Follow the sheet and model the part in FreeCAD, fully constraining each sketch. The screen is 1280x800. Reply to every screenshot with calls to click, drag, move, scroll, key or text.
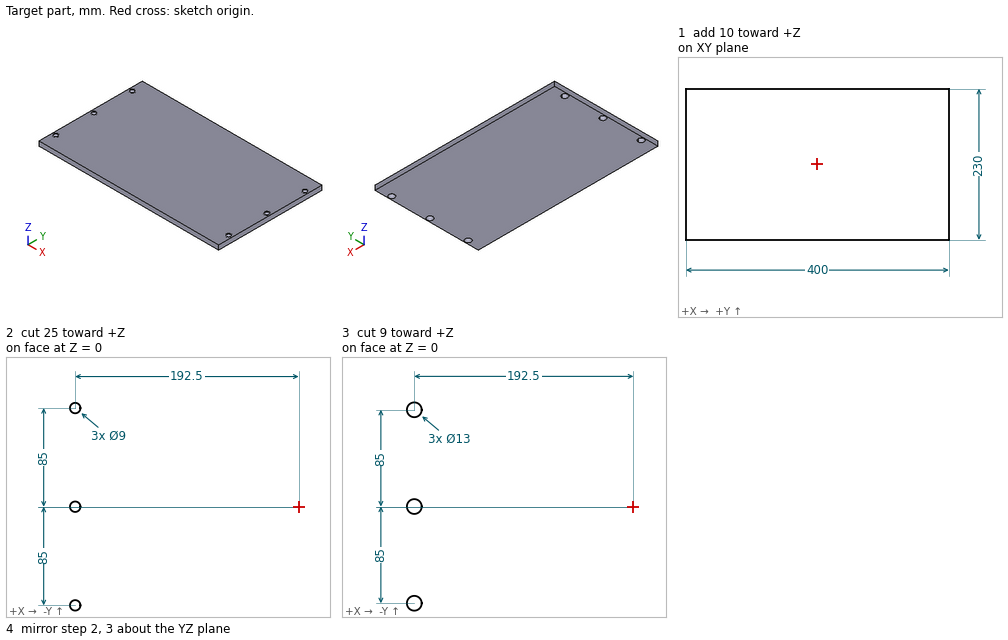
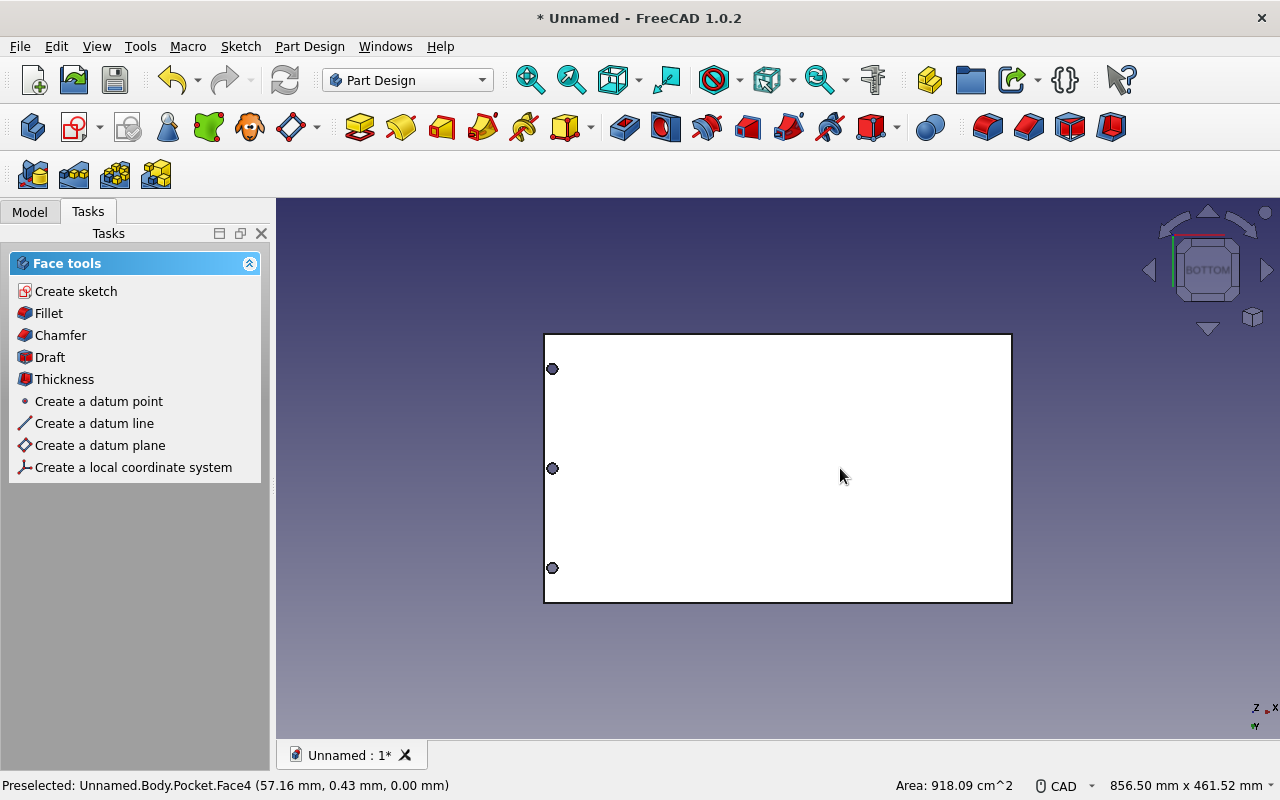
click(74, 128)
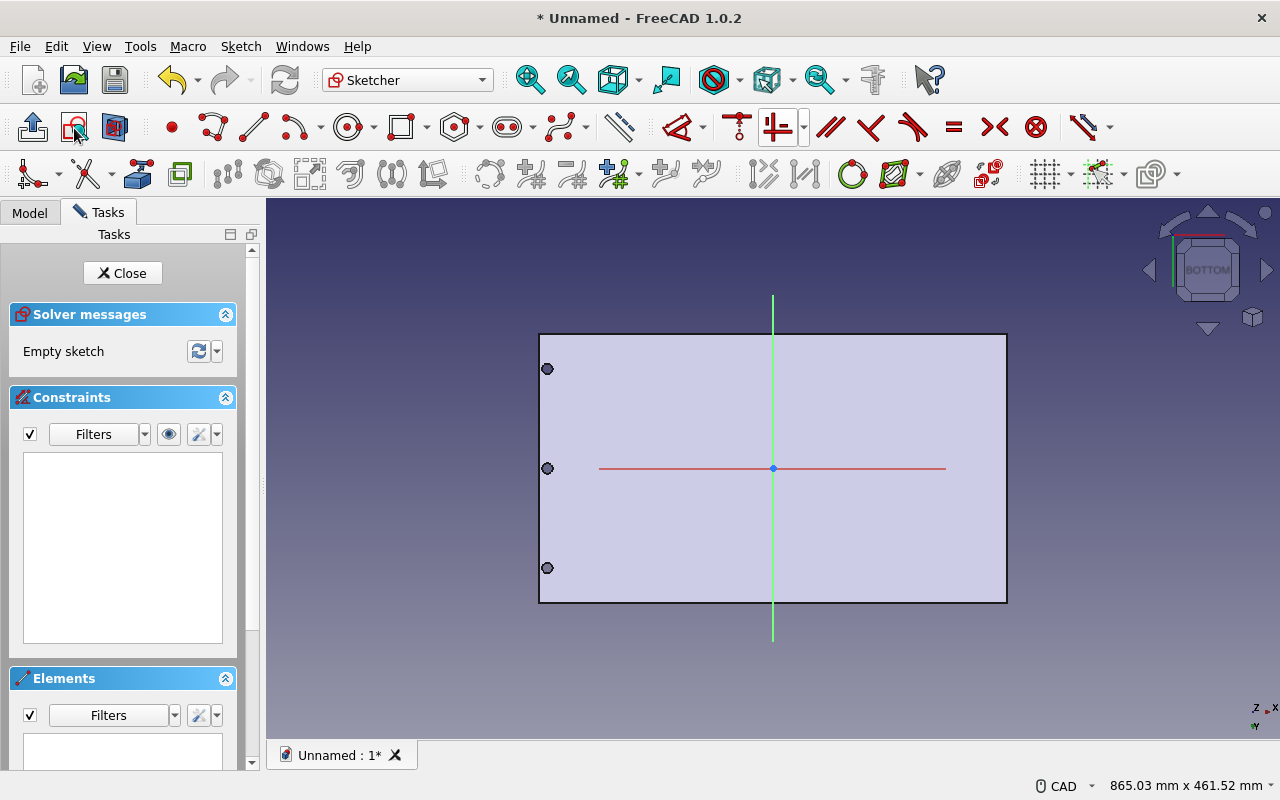
scroll(558, 469, up, 2)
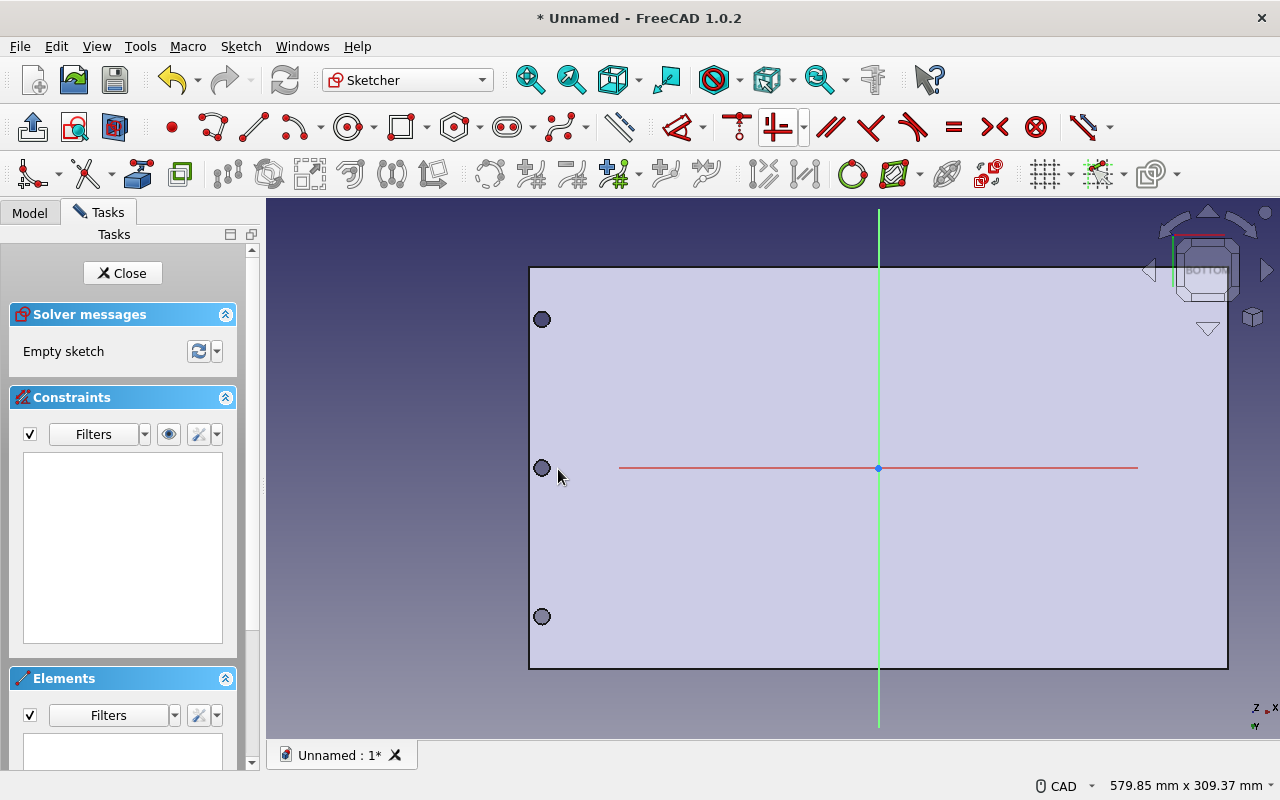
key(g)
key(c)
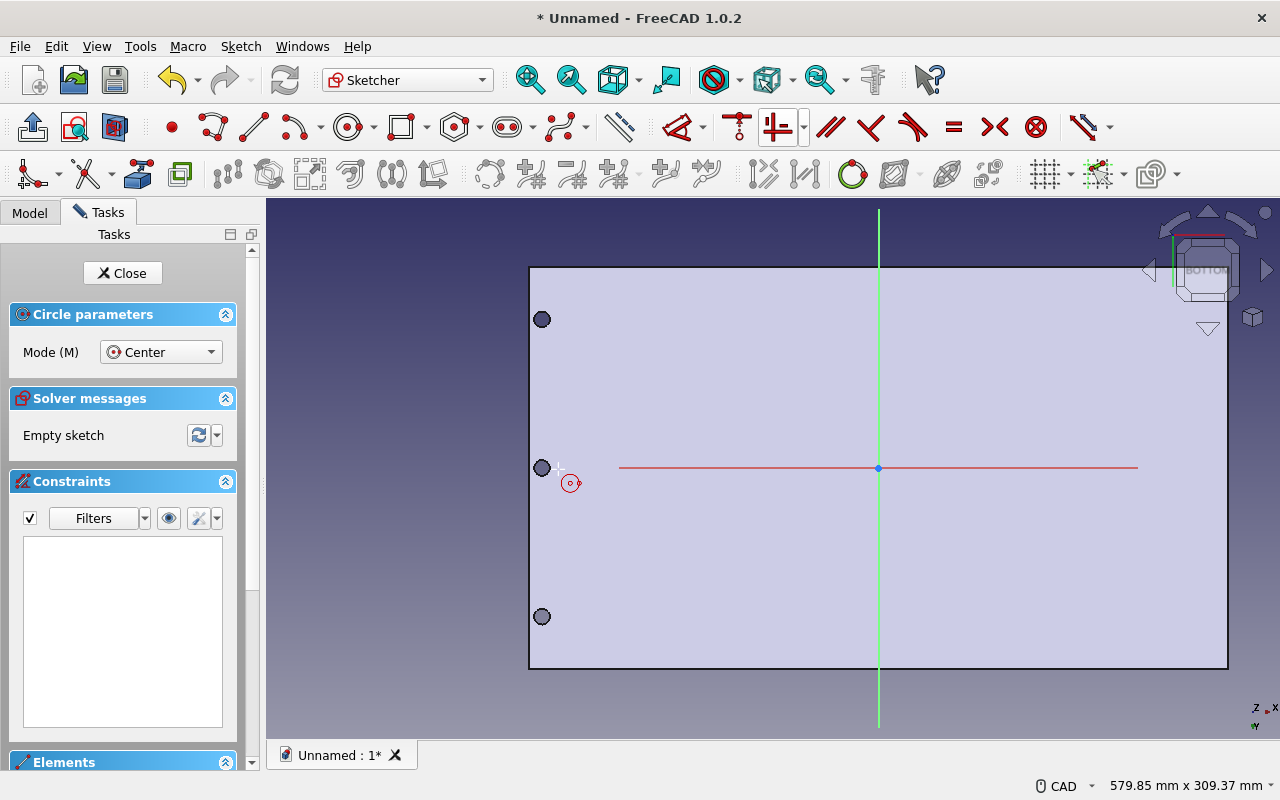
scroll(542, 319, up, 4)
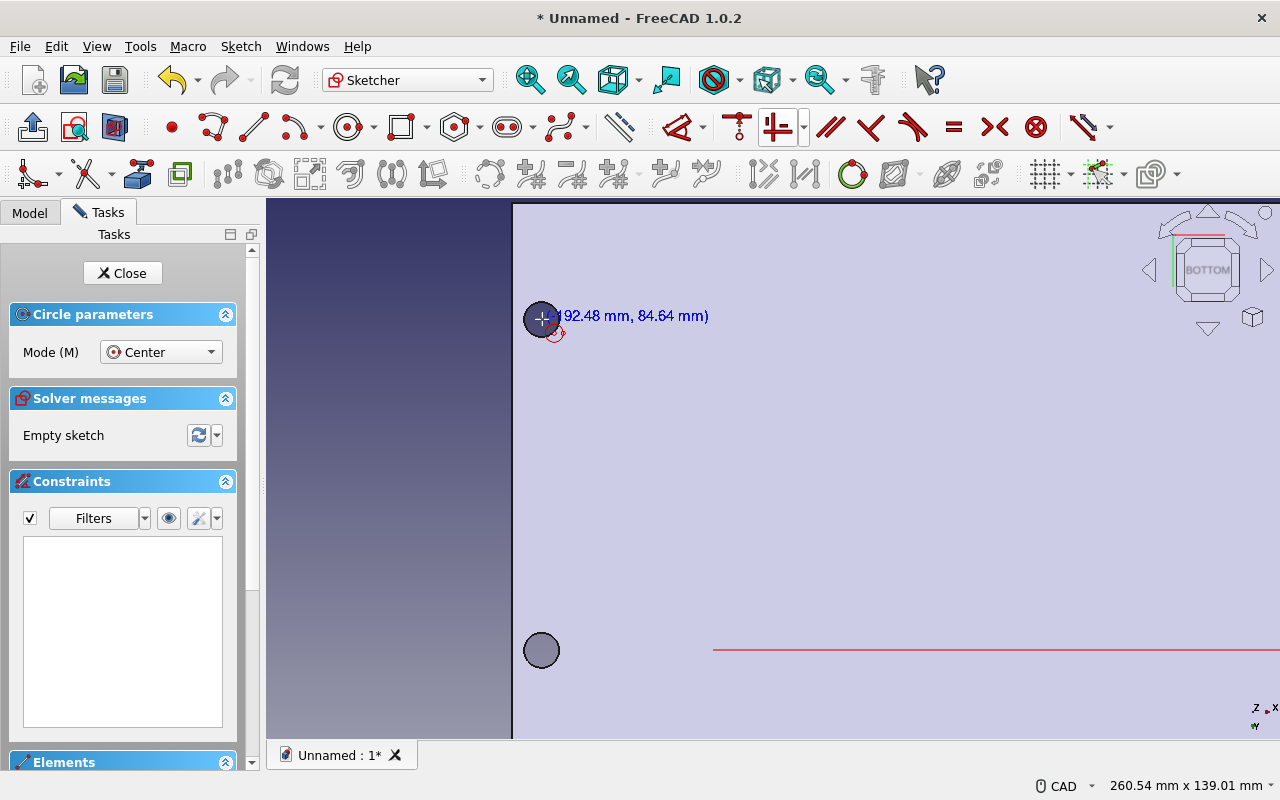
click(542, 320)
move(559, 302)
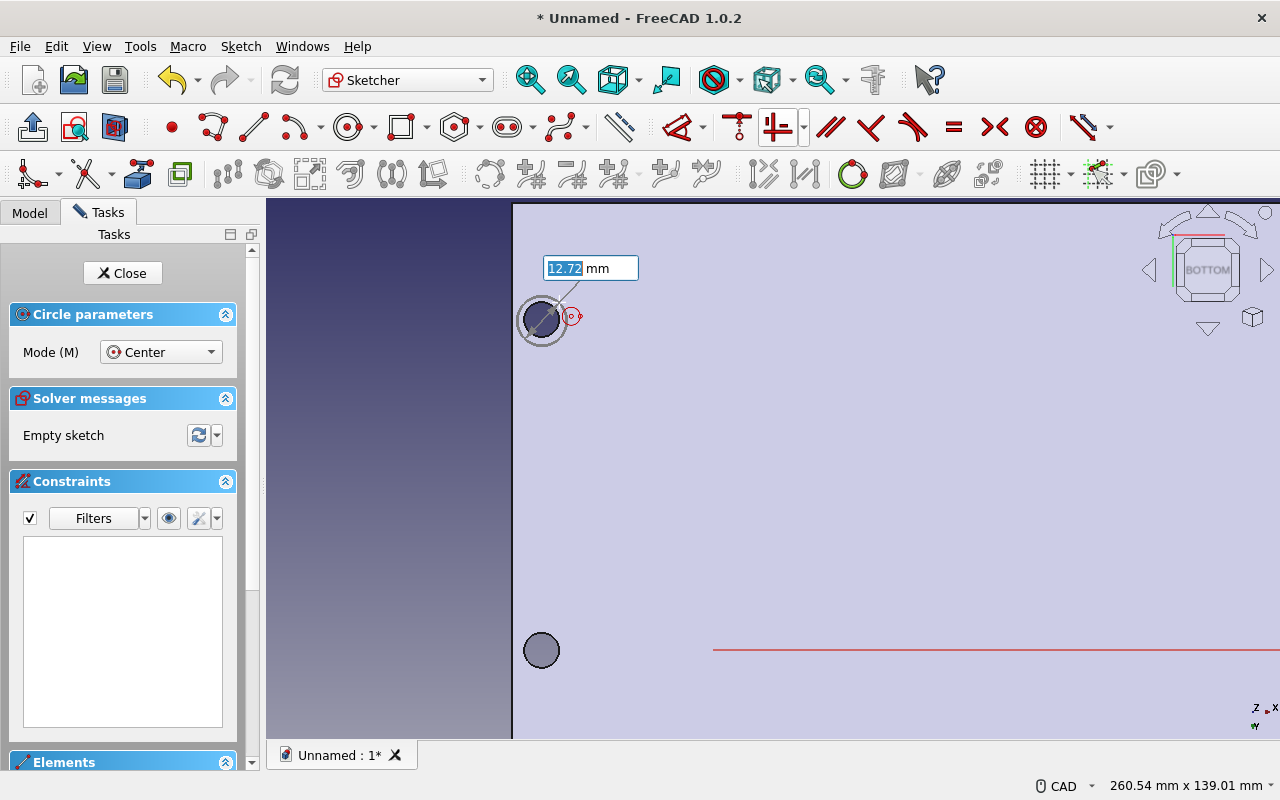
text(13)
key(Return)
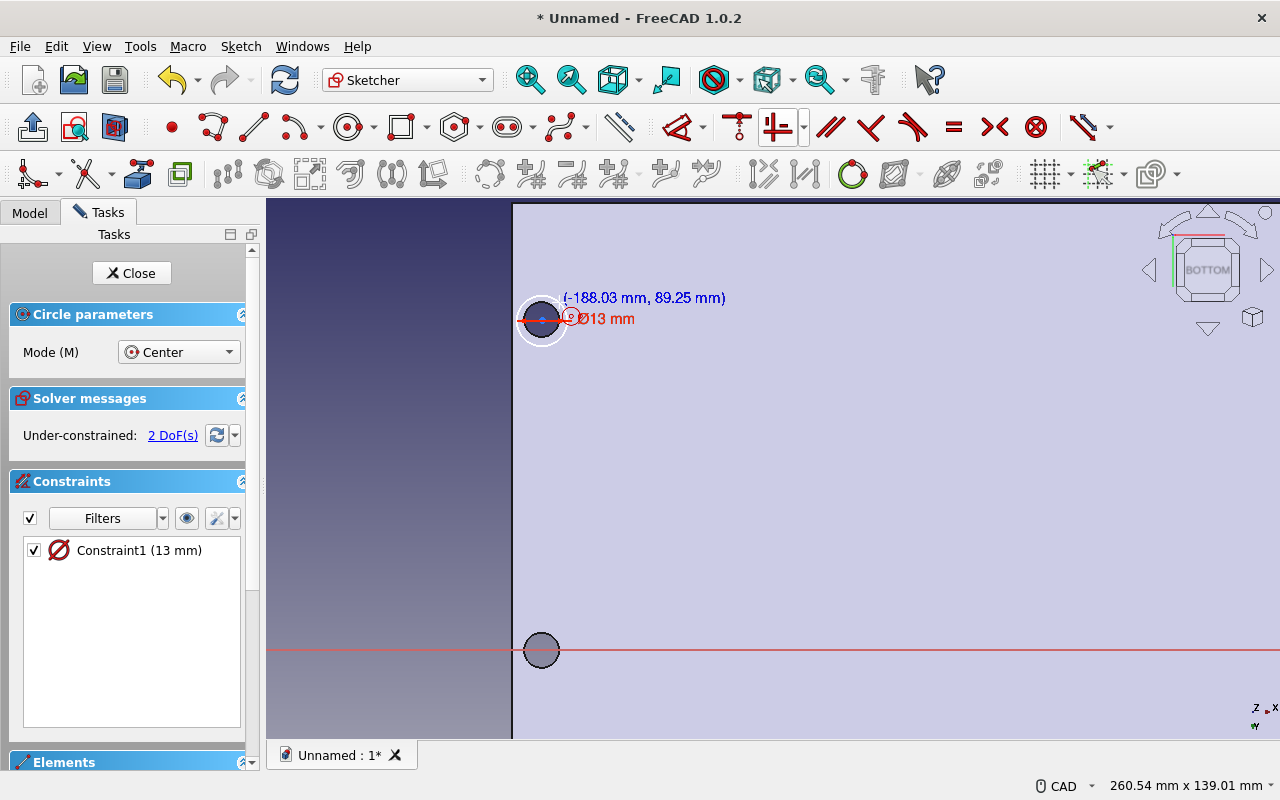
click(542, 650)
move(559, 632)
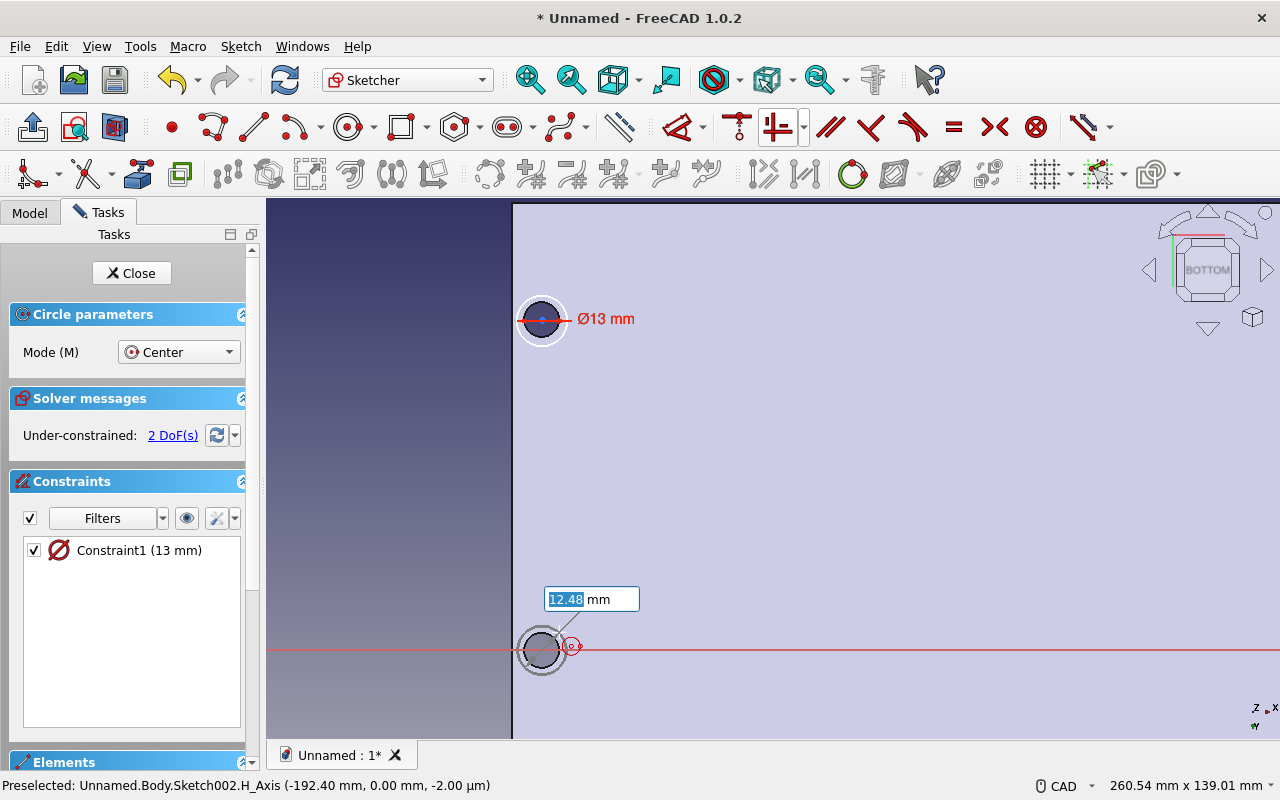
text(13)
key(Return)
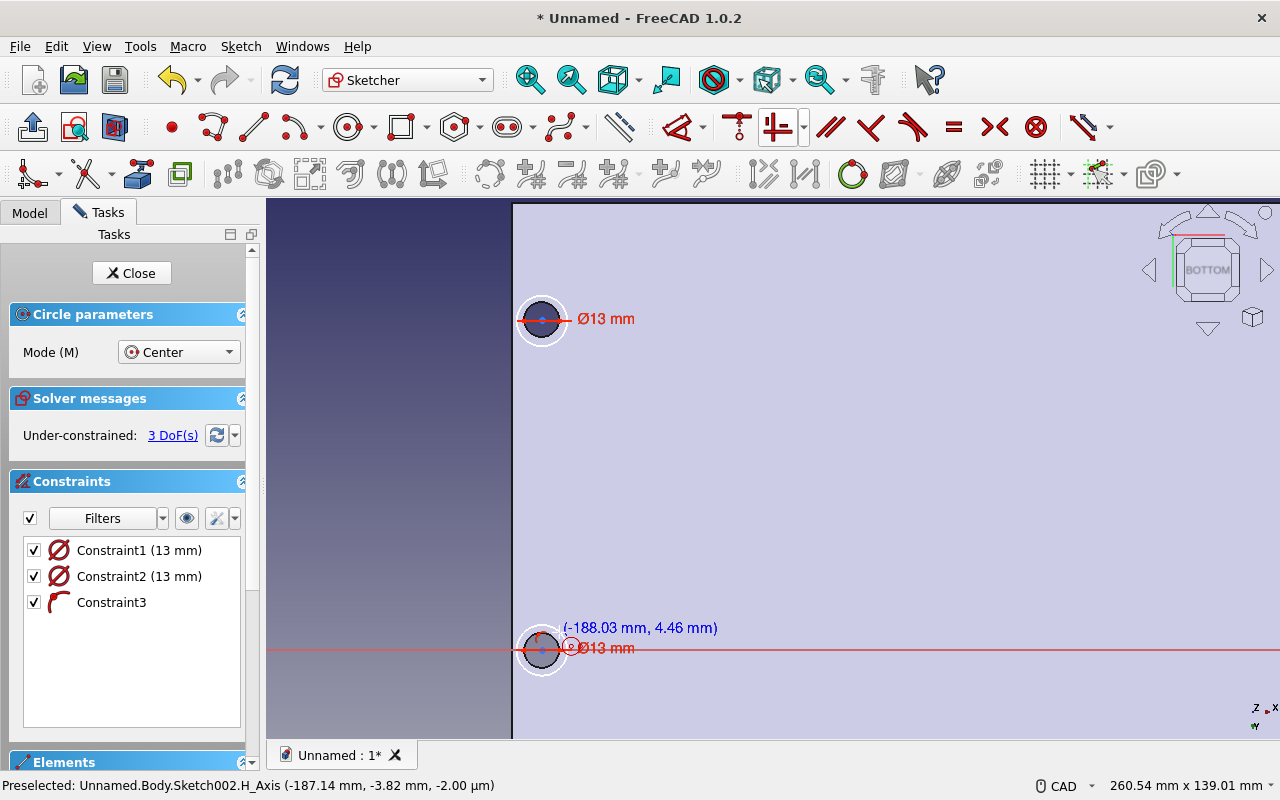
scroll(542, 320, down, 4)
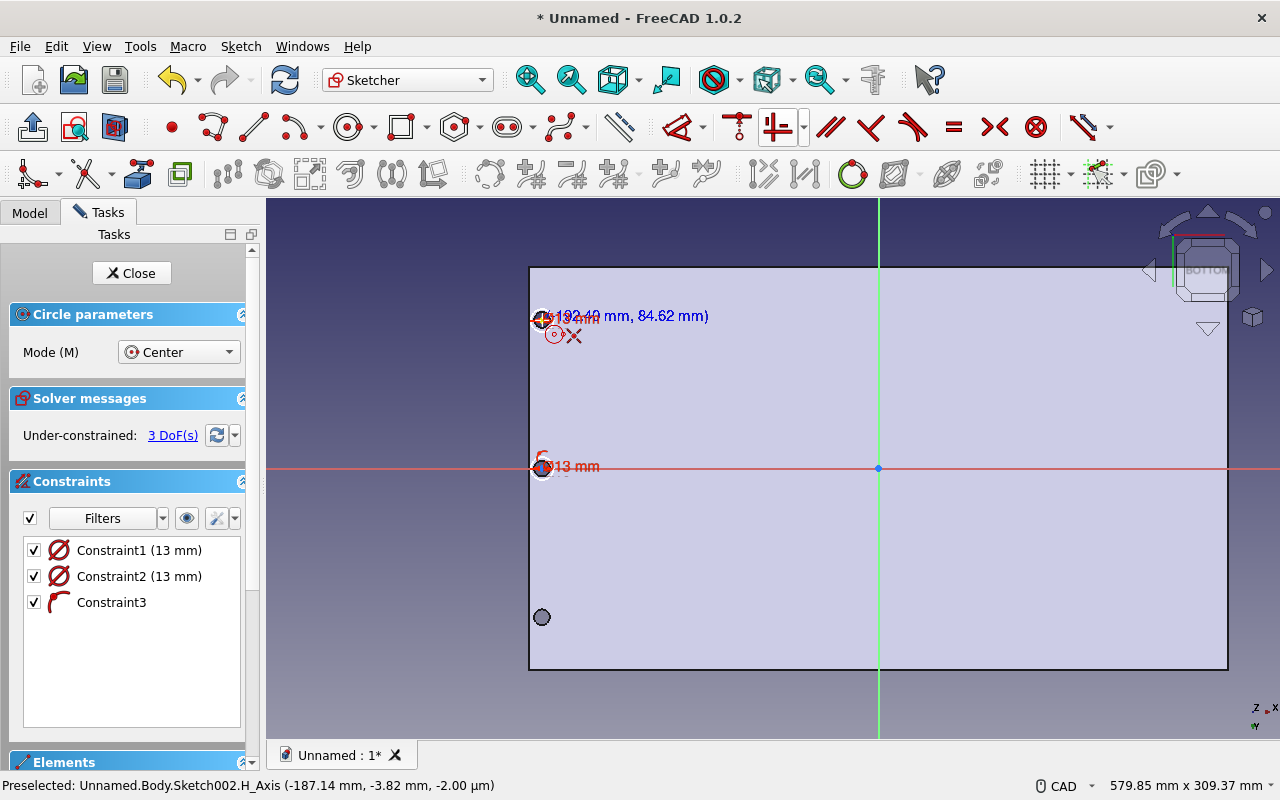
scroll(542, 617, up, 4)